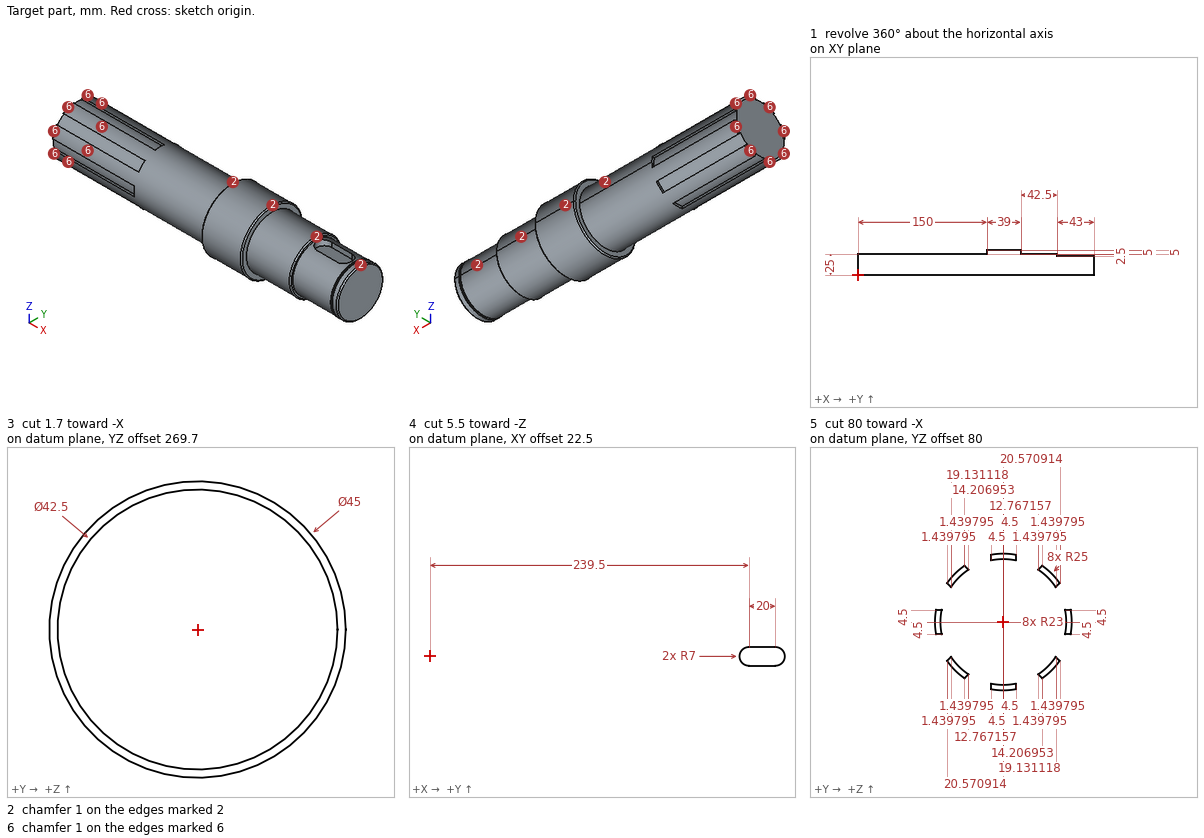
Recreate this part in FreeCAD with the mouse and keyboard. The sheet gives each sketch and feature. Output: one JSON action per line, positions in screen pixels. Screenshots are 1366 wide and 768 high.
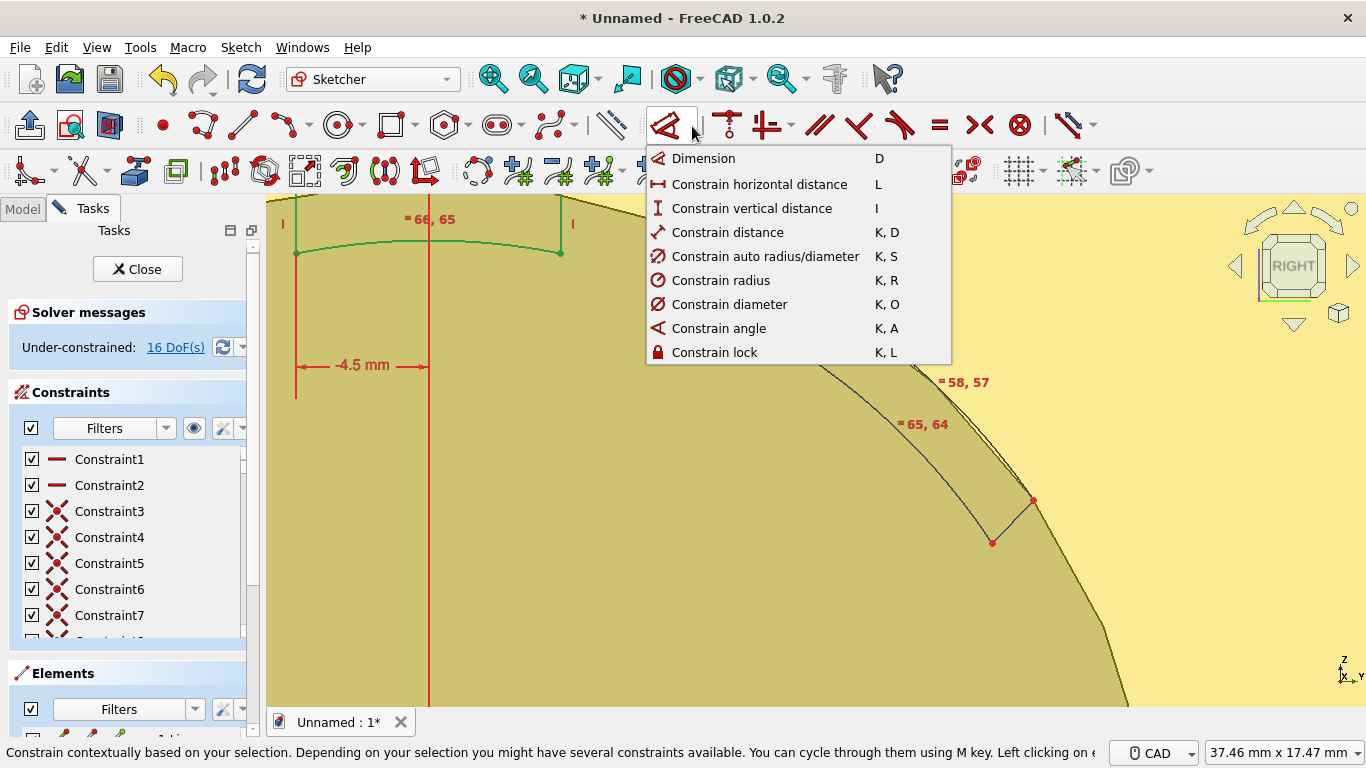
{"action": "left_click", "coordinate": [799, 184]}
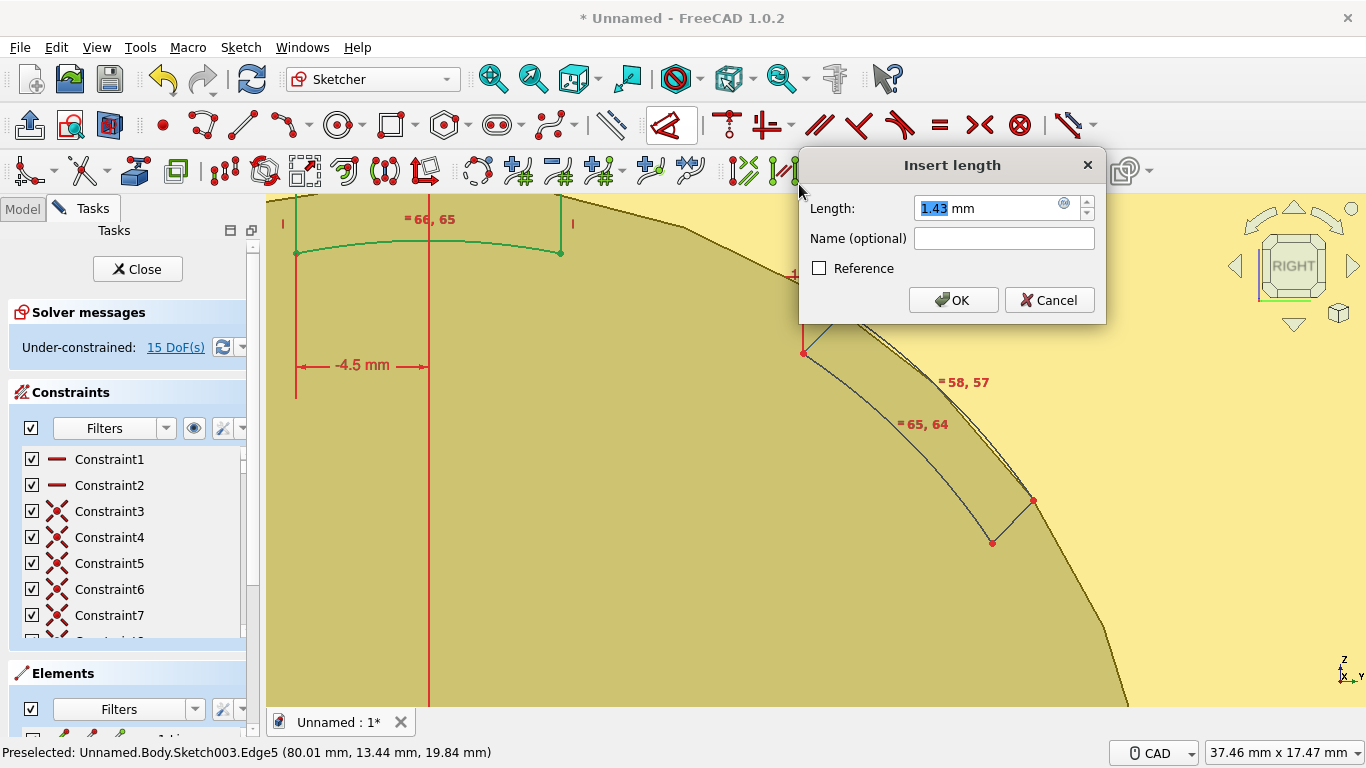
{"action": "type", "text": "1.439795"}
{"action": "key", "text": "Return"}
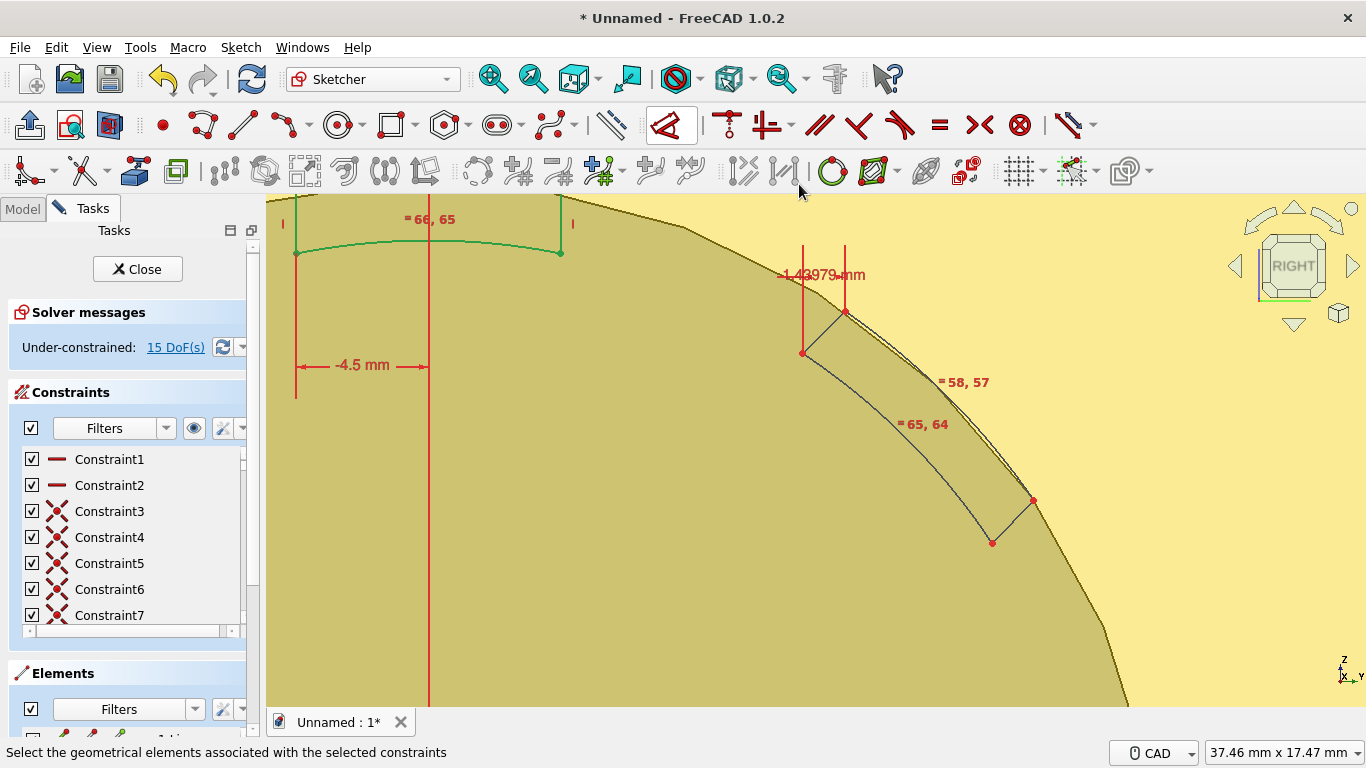
{"action": "left_click", "coordinate": [1021, 513]}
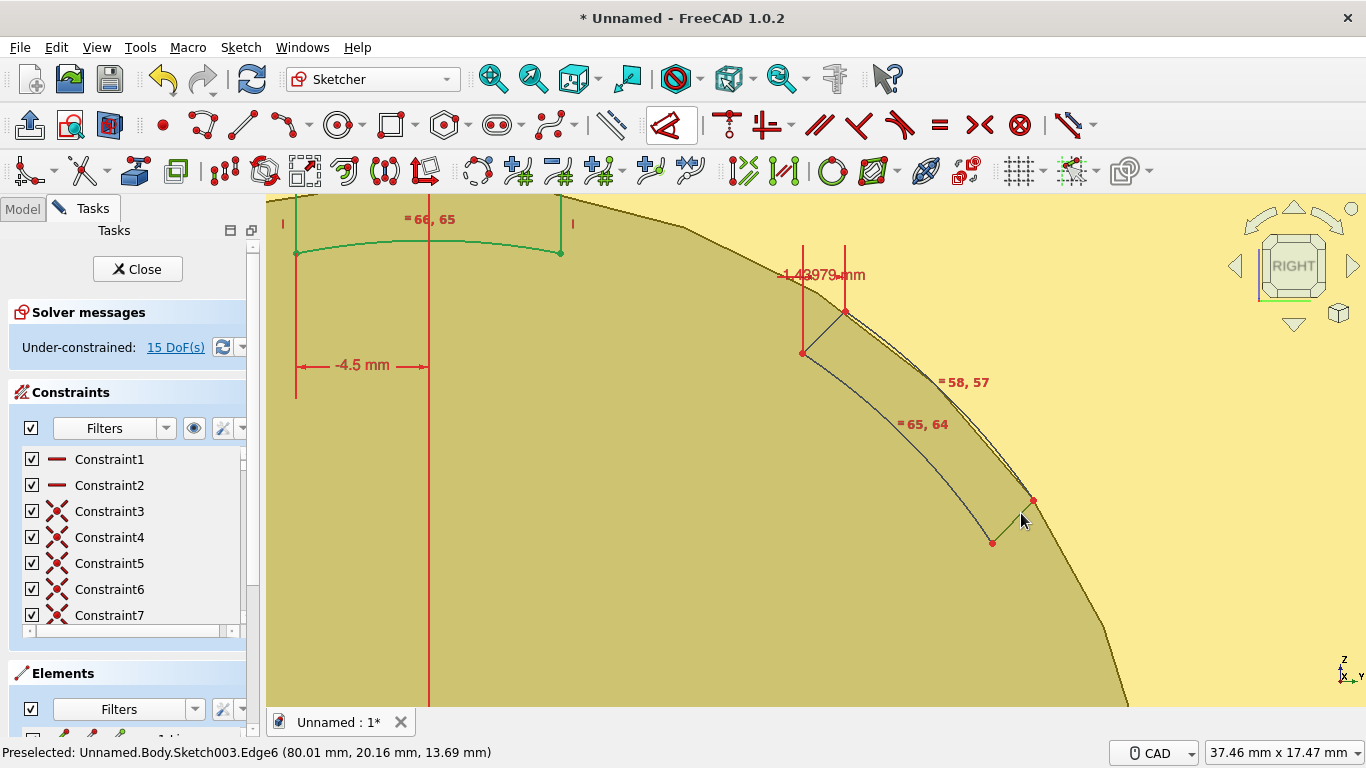
{"action": "key", "text": "l"}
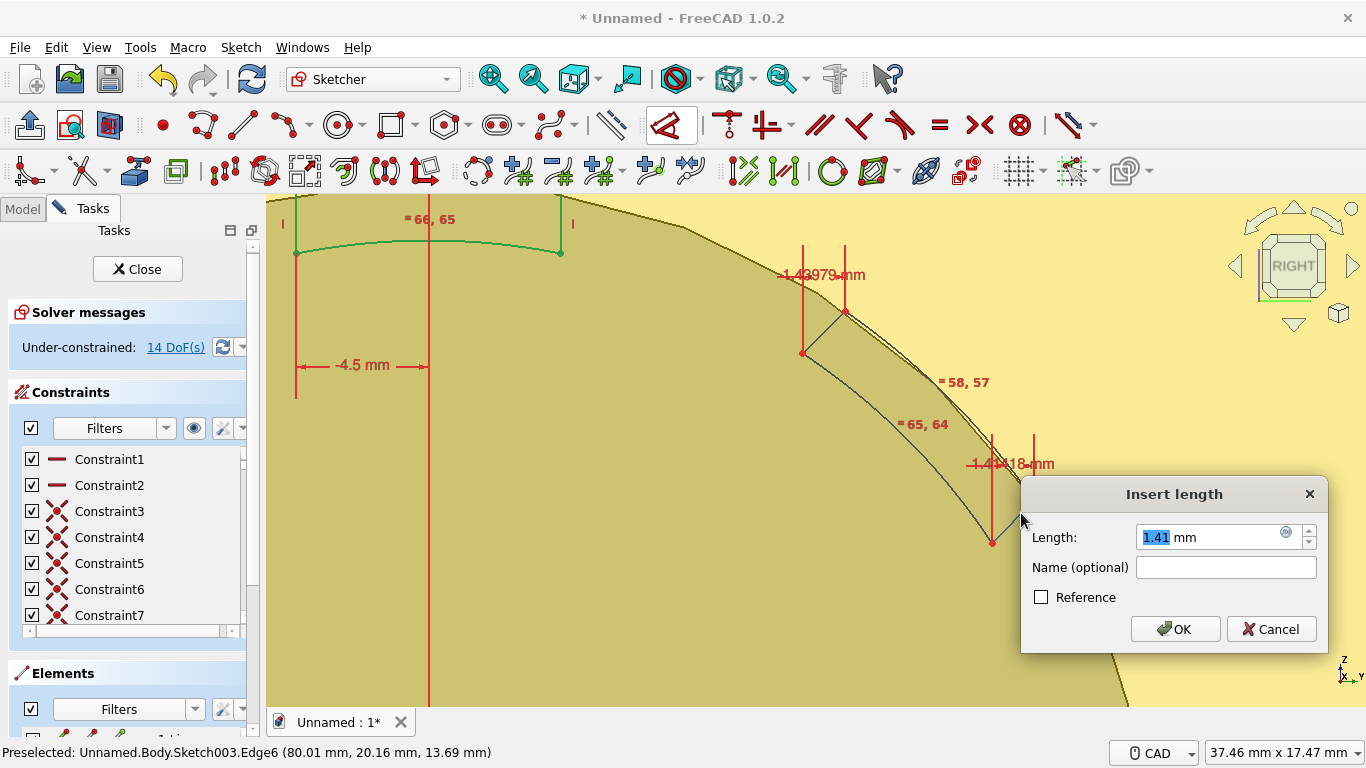
{"action": "type", "text": "1.439795"}
{"action": "key", "text": "Return"}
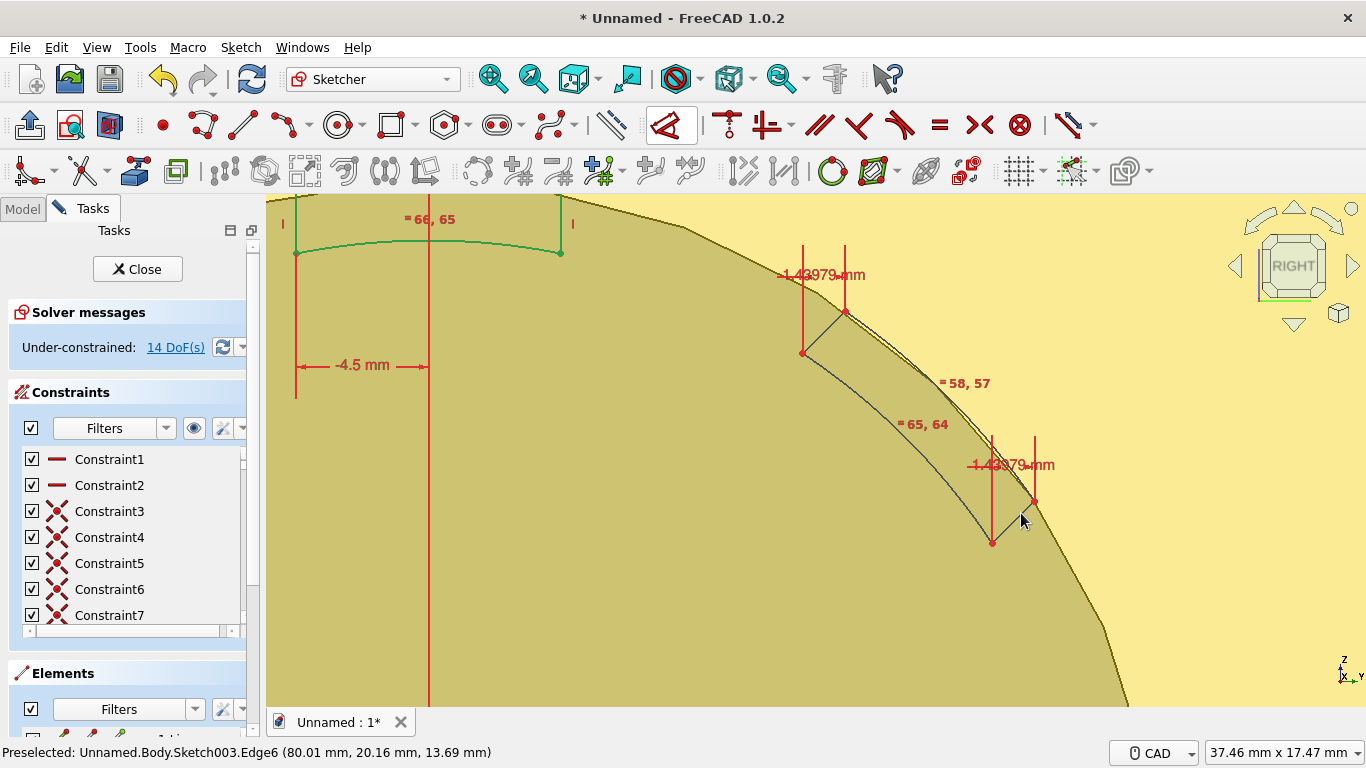
{"action": "scroll", "coordinate": [828, 333], "scroll_direction": "down", "scroll_amount": 8}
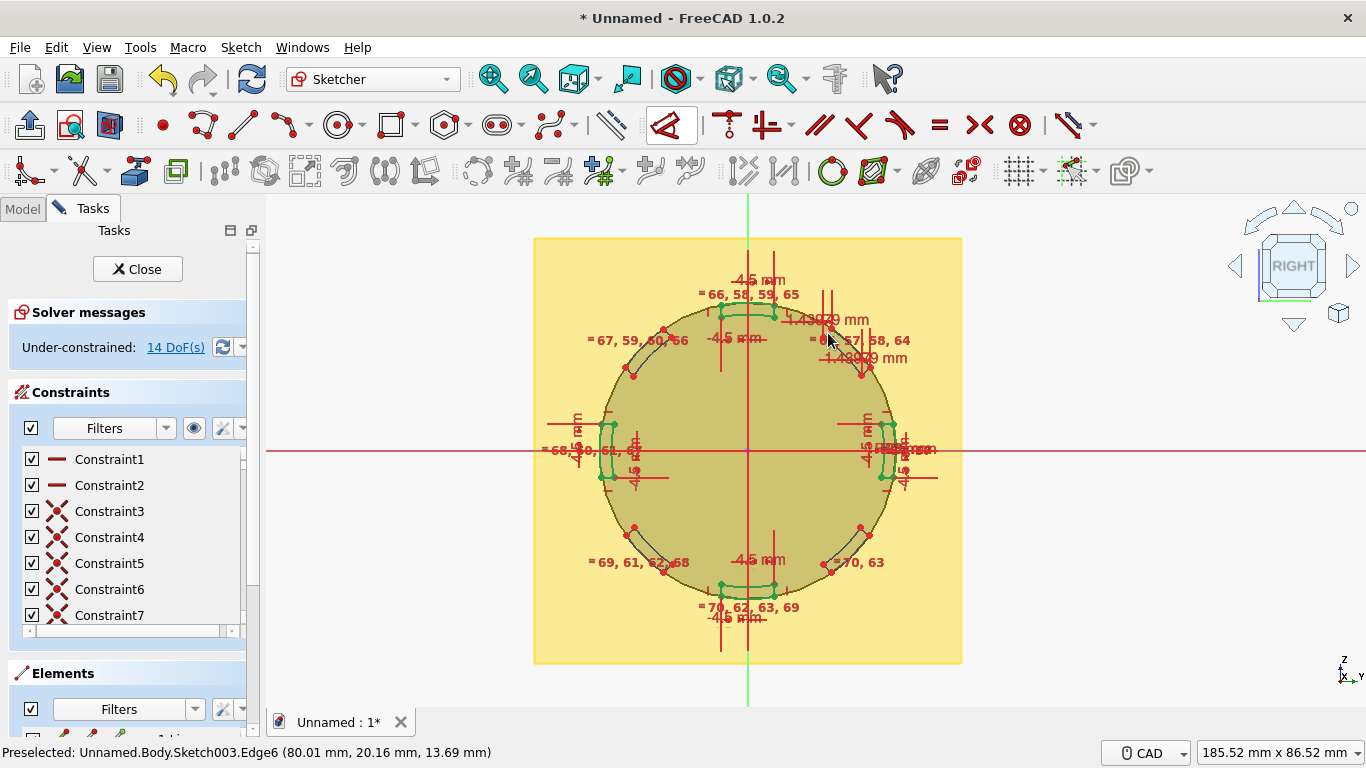
{"action": "scroll", "coordinate": [631, 374], "scroll_direction": "up", "scroll_amount": 8}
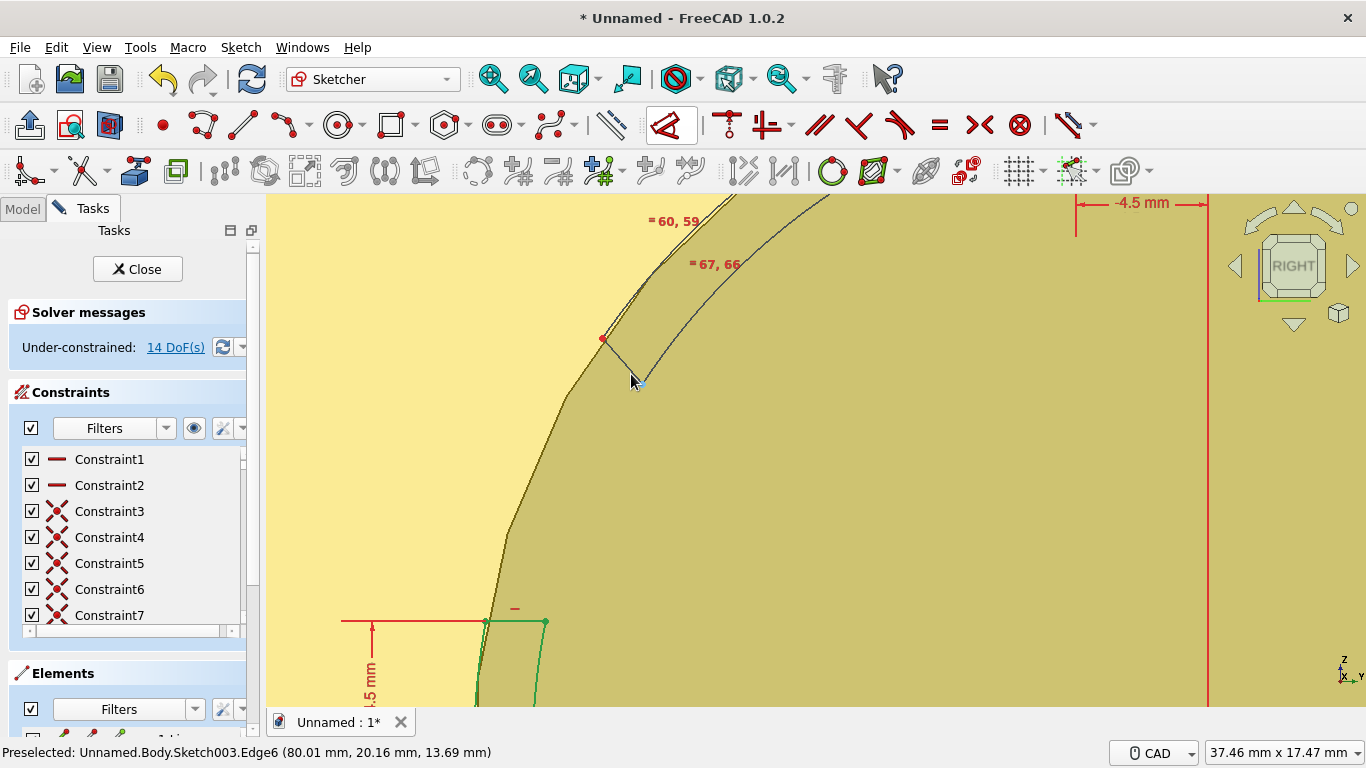
{"action": "left_click", "coordinate": [631, 370]}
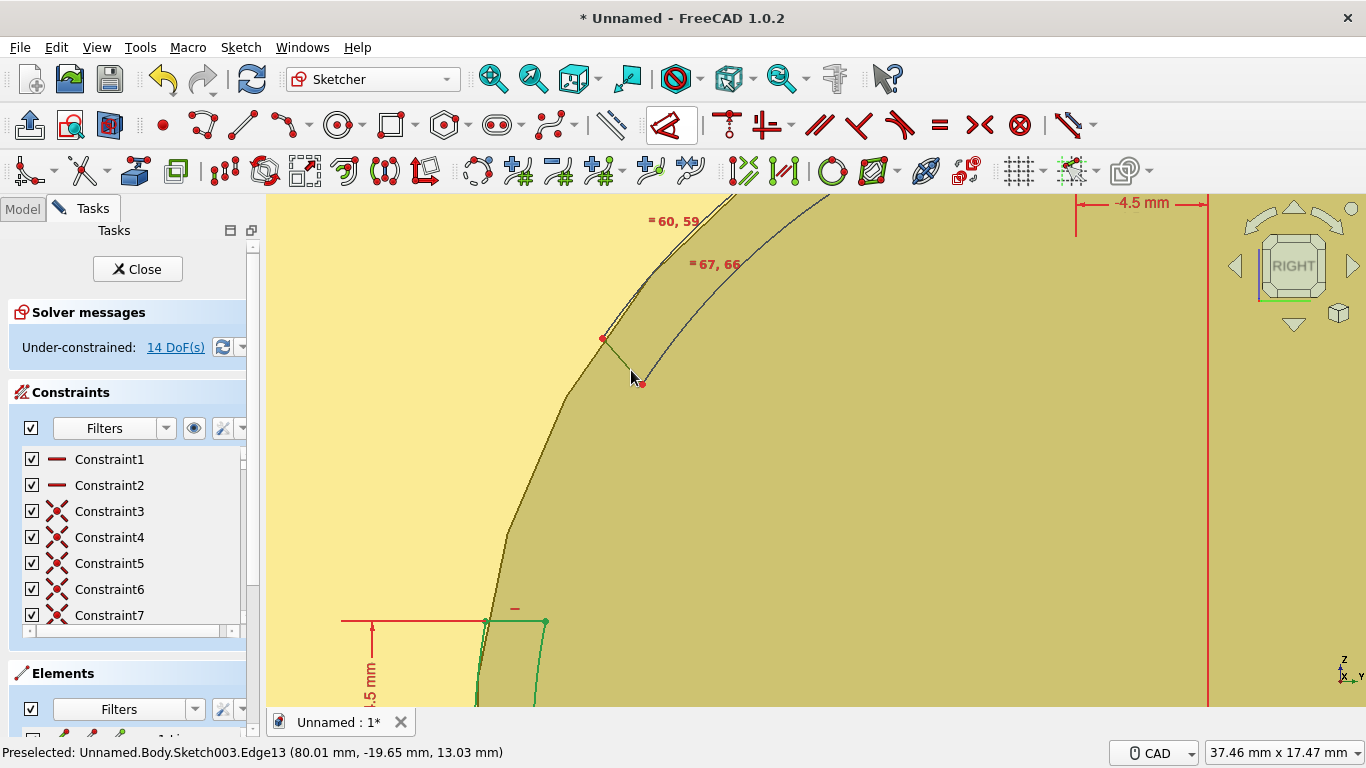
{"action": "key", "text": "l"}